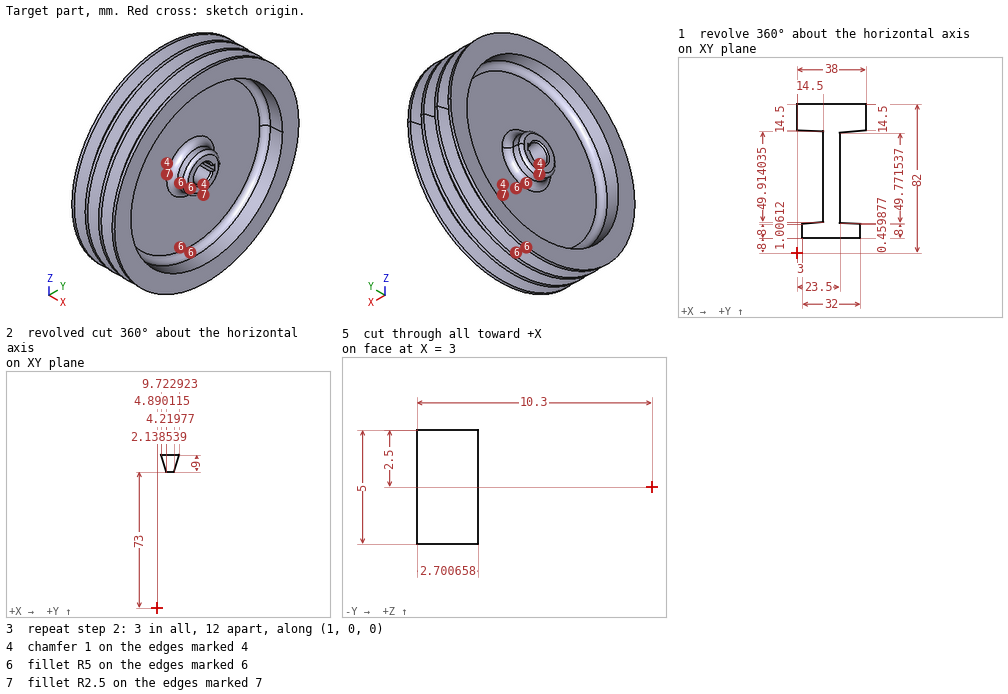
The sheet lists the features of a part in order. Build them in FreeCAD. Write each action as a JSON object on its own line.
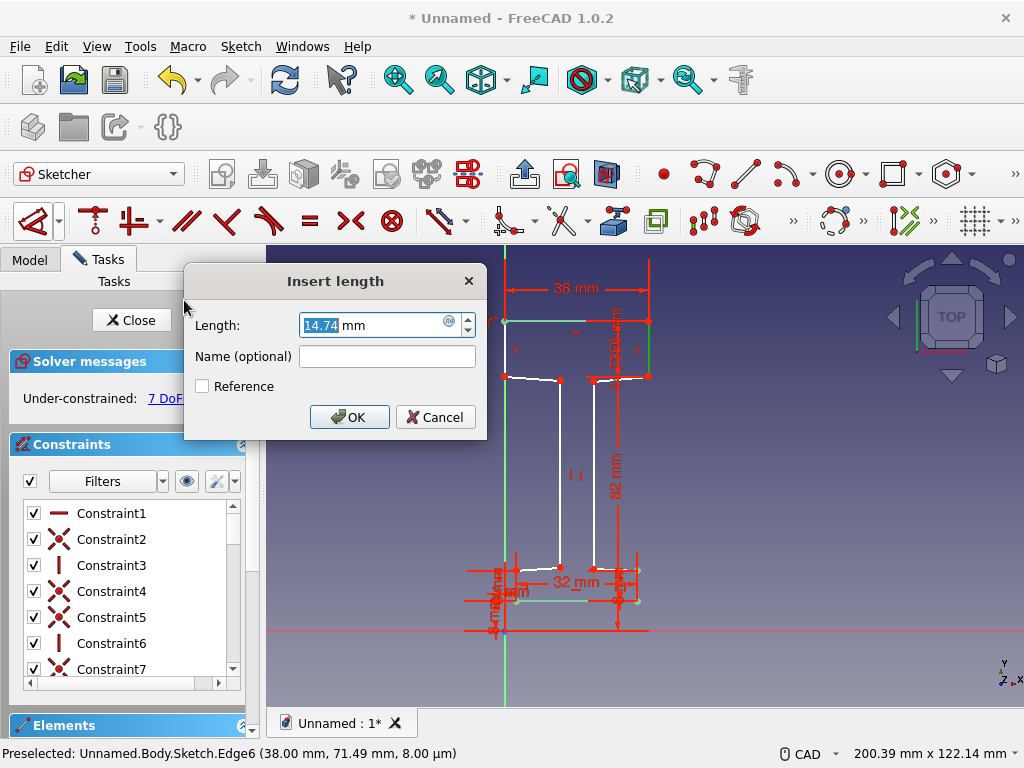
{"action": "type", "text": "14.5"}
{"action": "key", "text": "Return"}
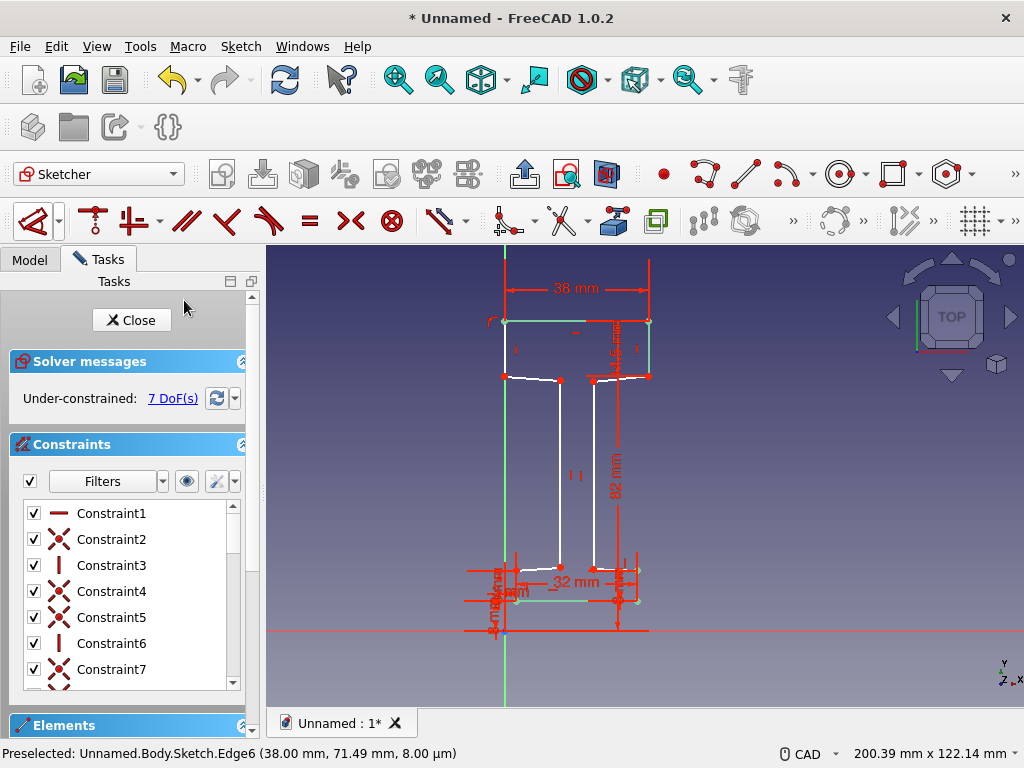
{"action": "left_click", "coordinate": [505, 338]}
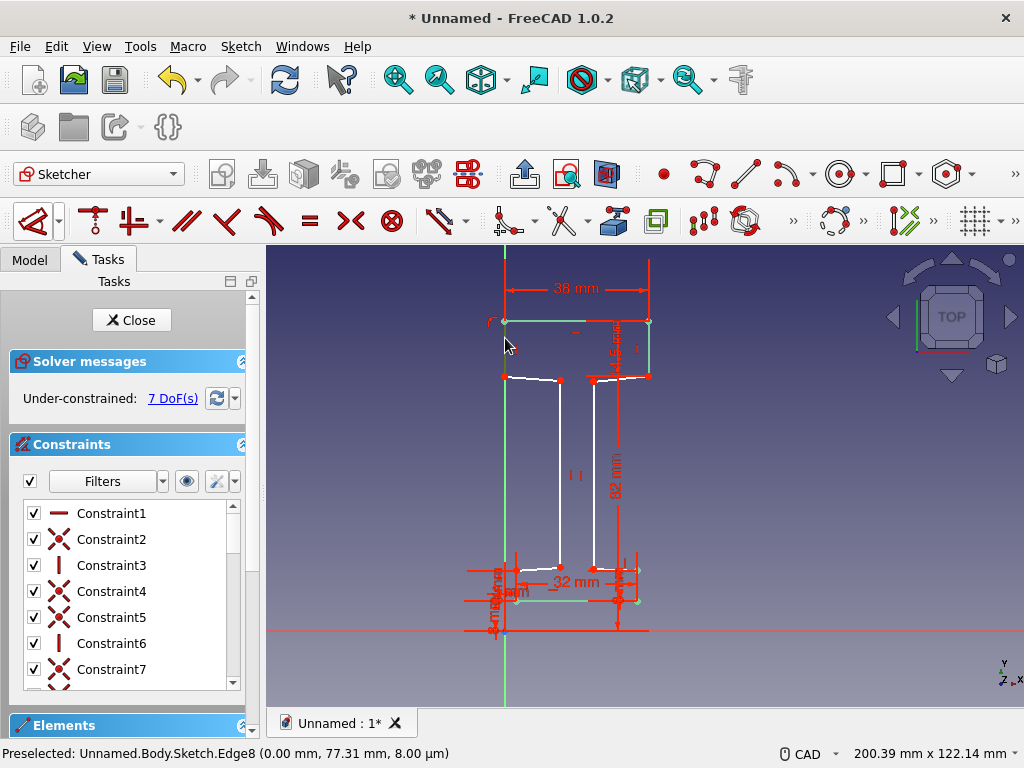
{"action": "left_click", "coordinate": [58, 222]}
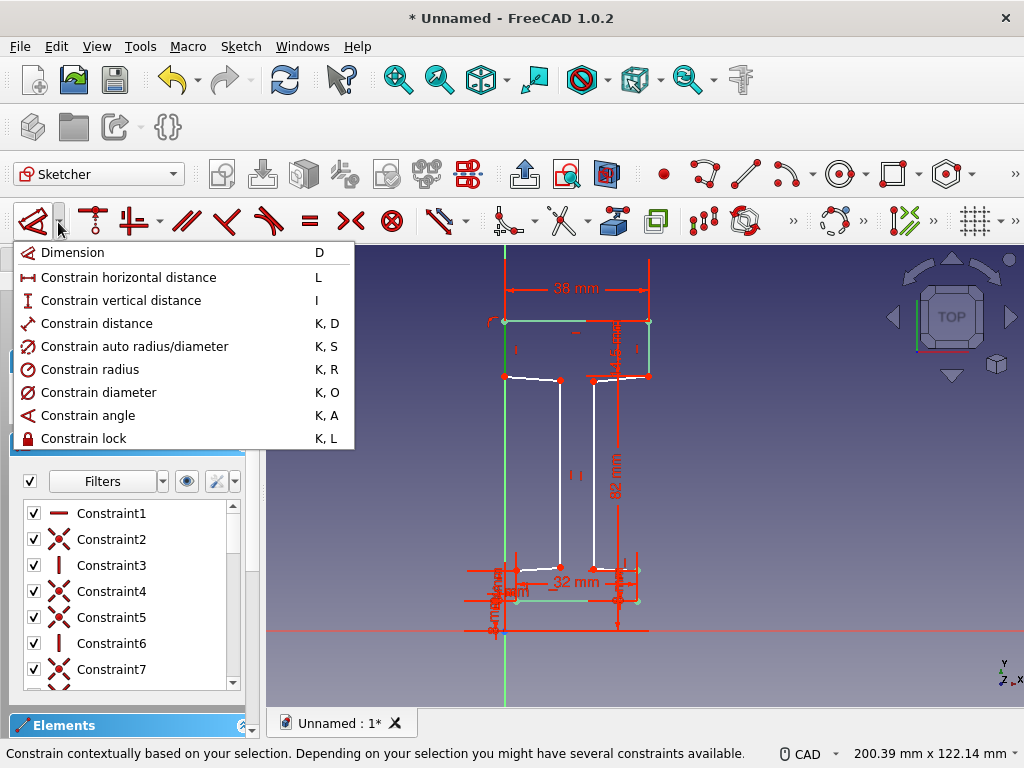
{"action": "left_click", "coordinate": [184, 300]}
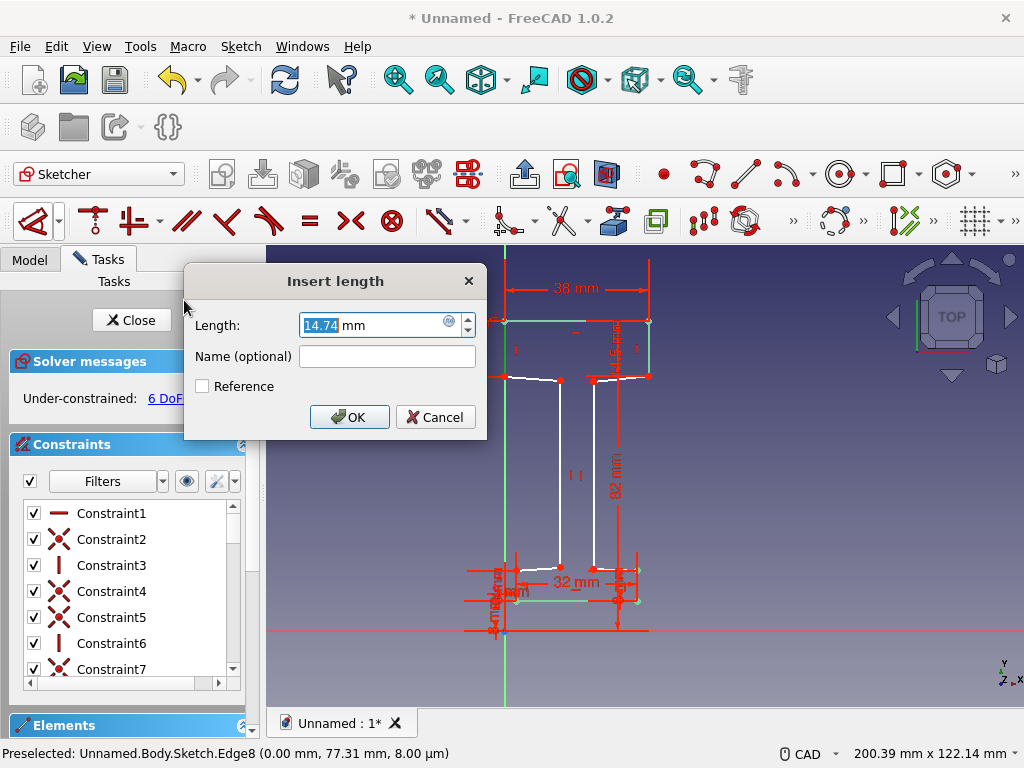
{"action": "type", "text": "14.5"}
{"action": "key", "text": "Return"}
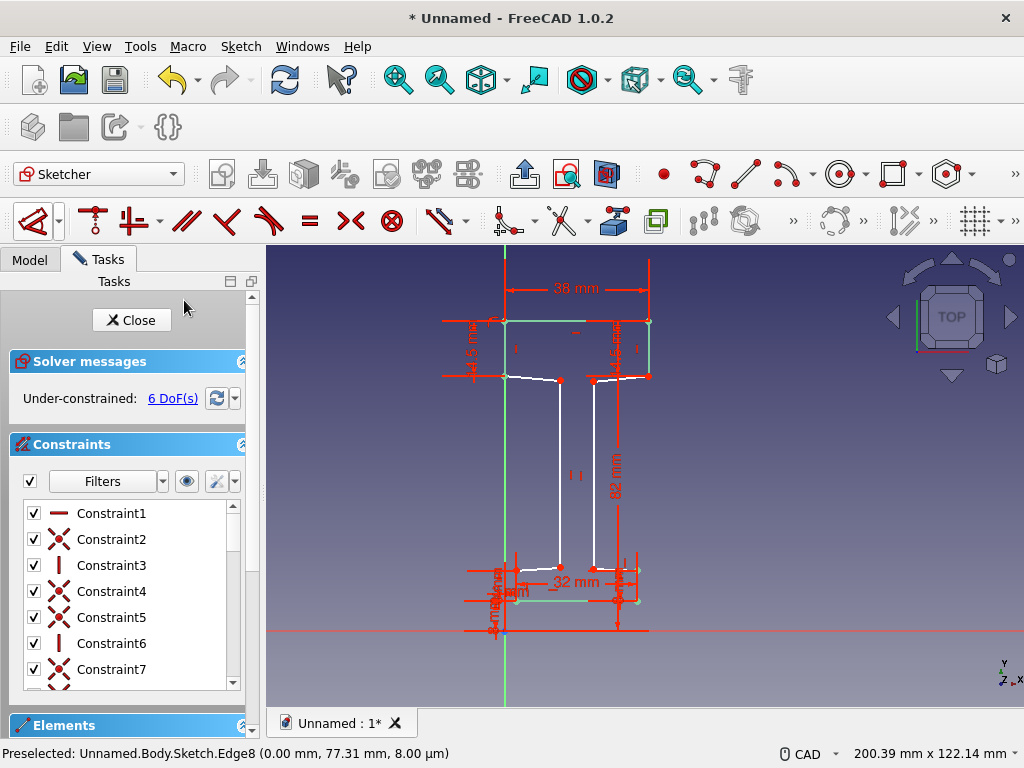
{"action": "left_click", "coordinate": [594, 569]}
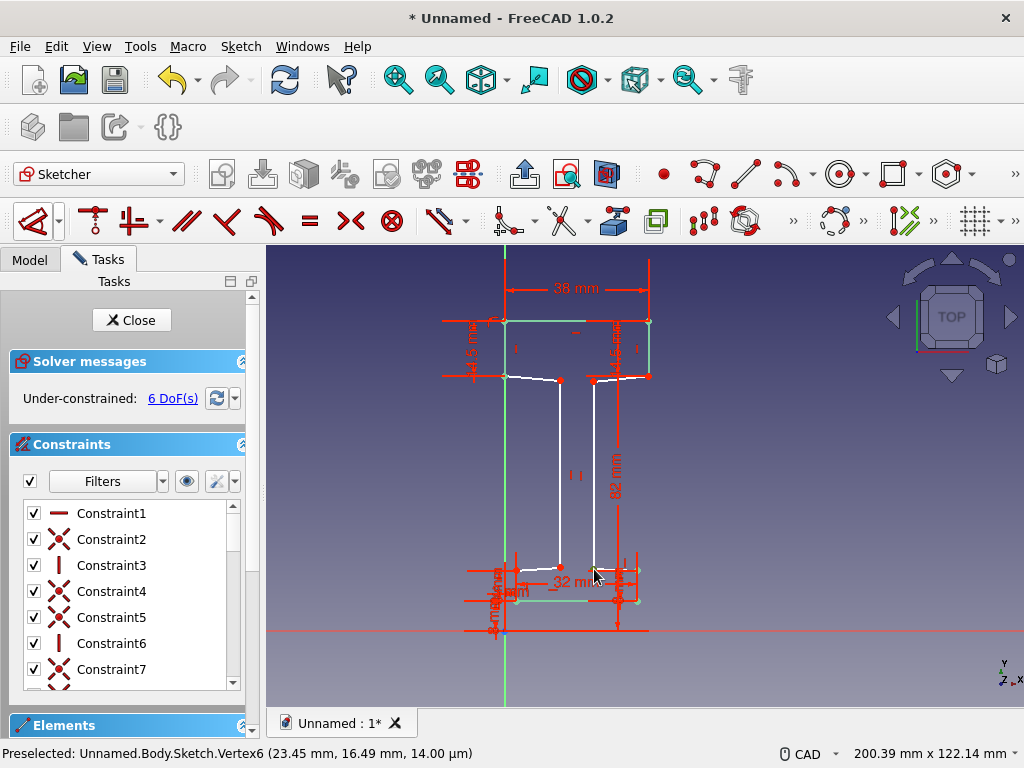
{"action": "key", "text": "l"}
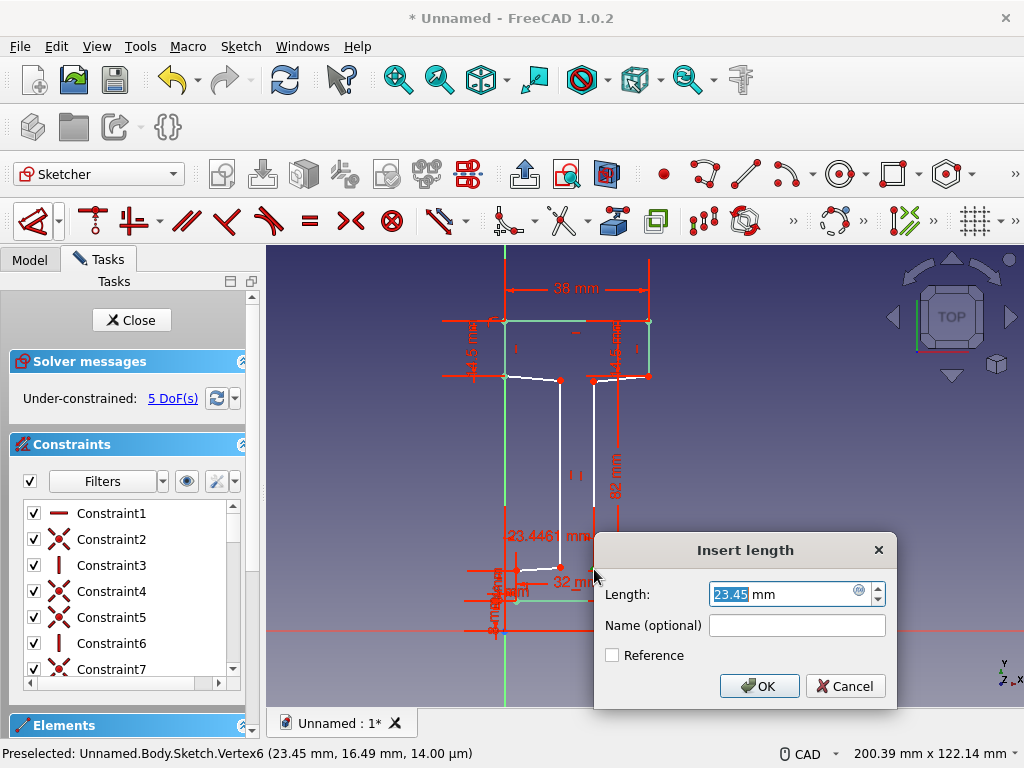
{"action": "type", "text": "23.5"}
{"action": "key", "text": "Return"}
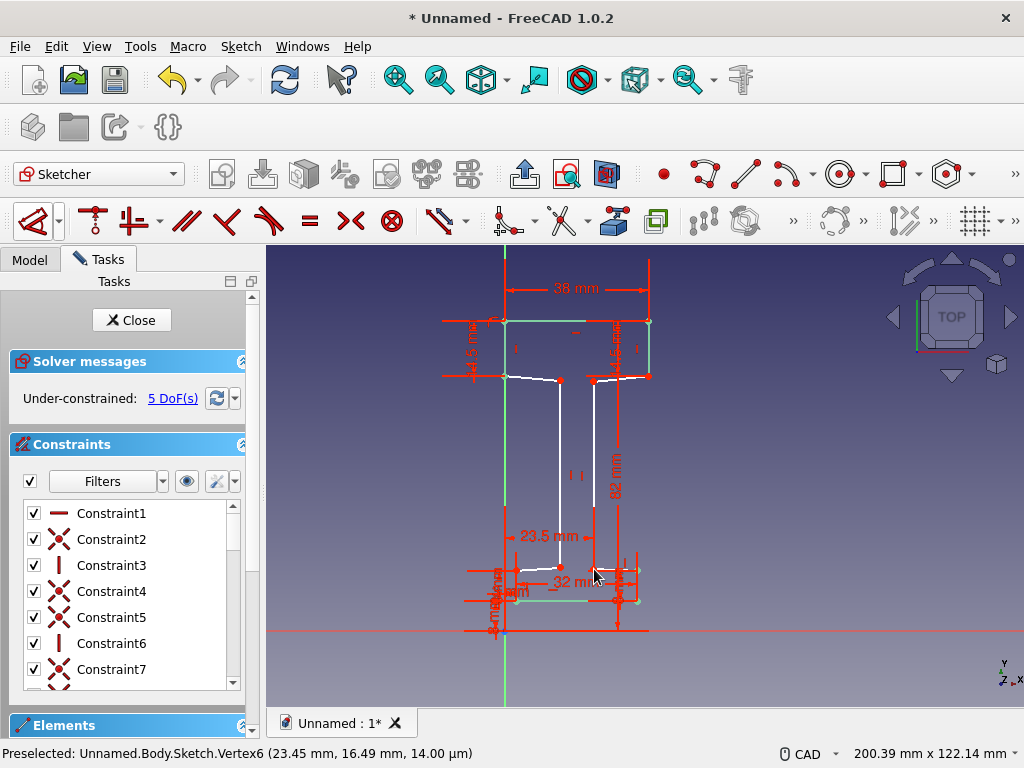
{"action": "left_click", "coordinate": [560, 381]}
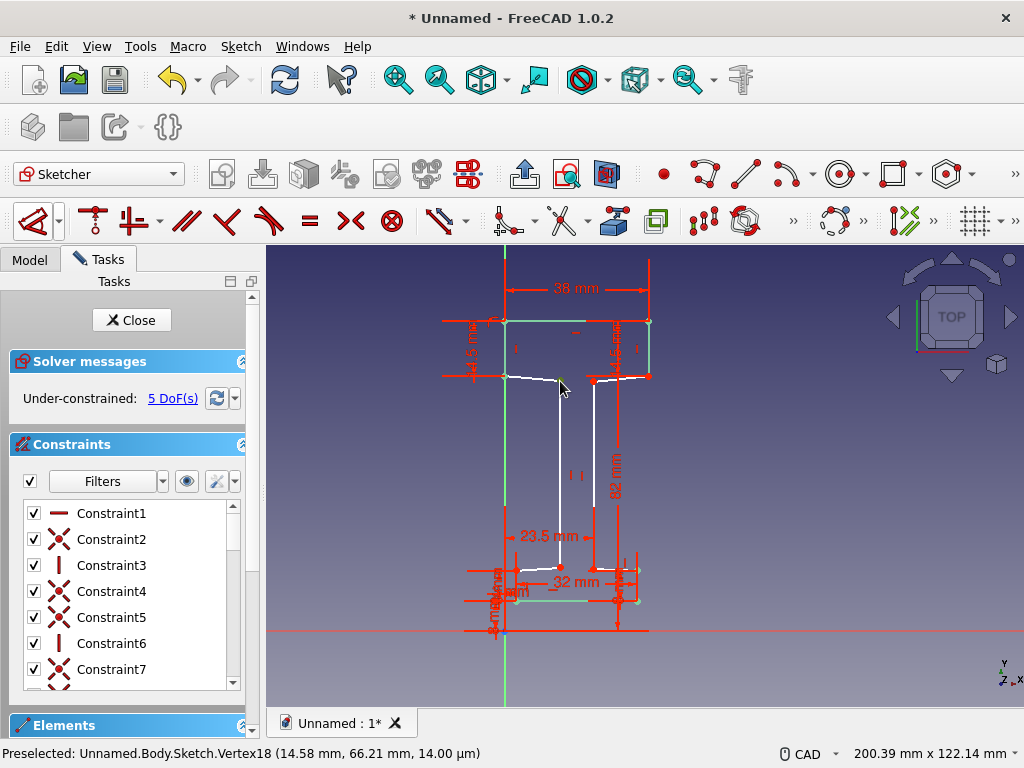
{"action": "key", "text": "l"}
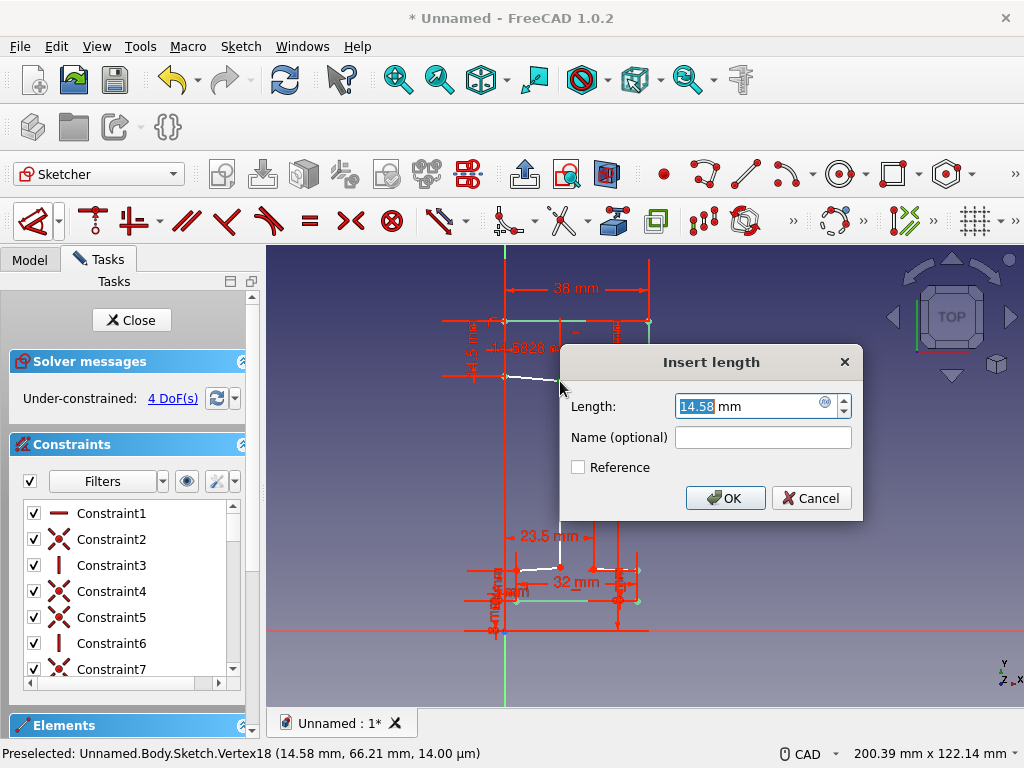
{"action": "type", "text": "14.5"}
{"action": "key", "text": "Return"}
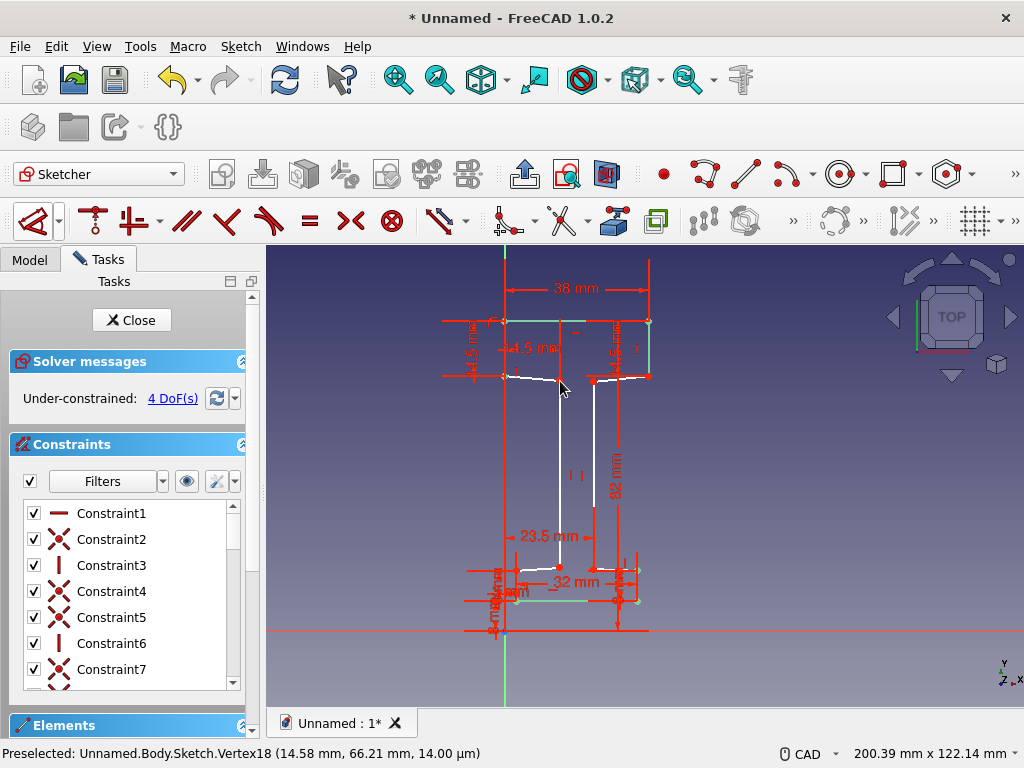
{"action": "scroll", "coordinate": [547, 569], "scroll_direction": "up", "scroll_amount": 12}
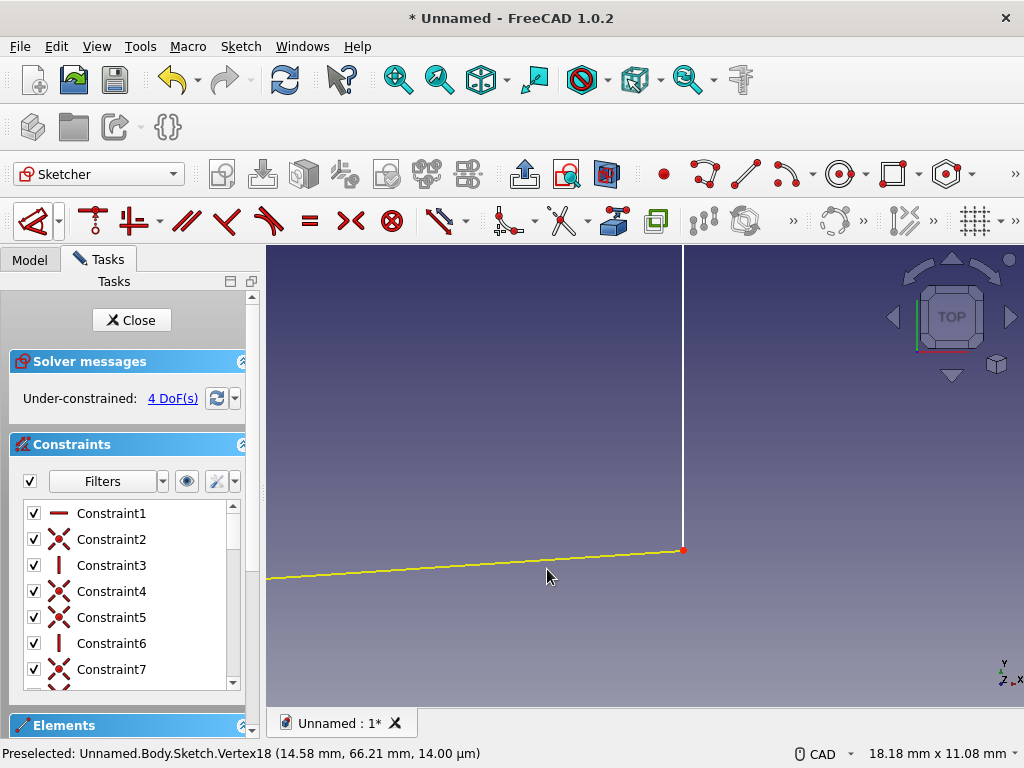
{"action": "left_click", "coordinate": [539, 561]}